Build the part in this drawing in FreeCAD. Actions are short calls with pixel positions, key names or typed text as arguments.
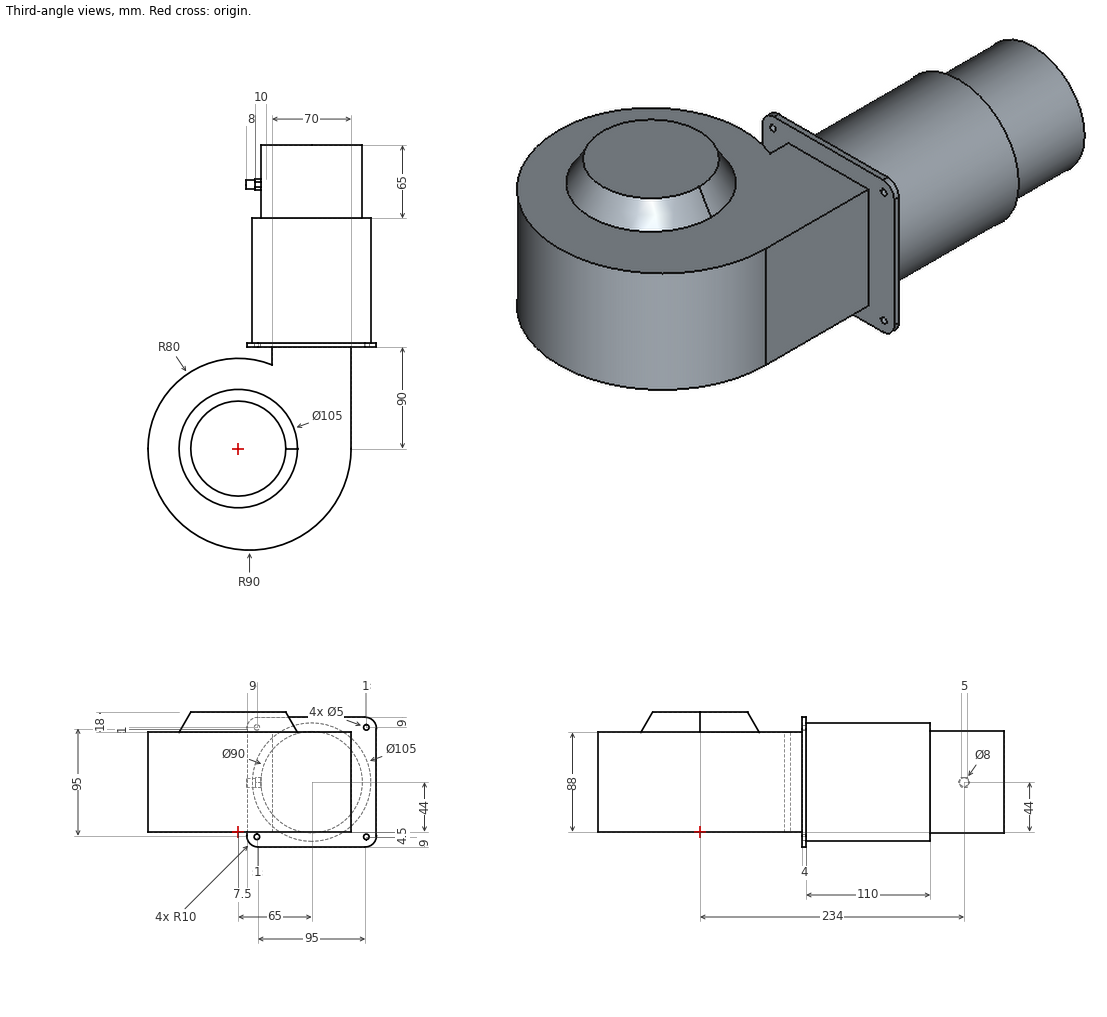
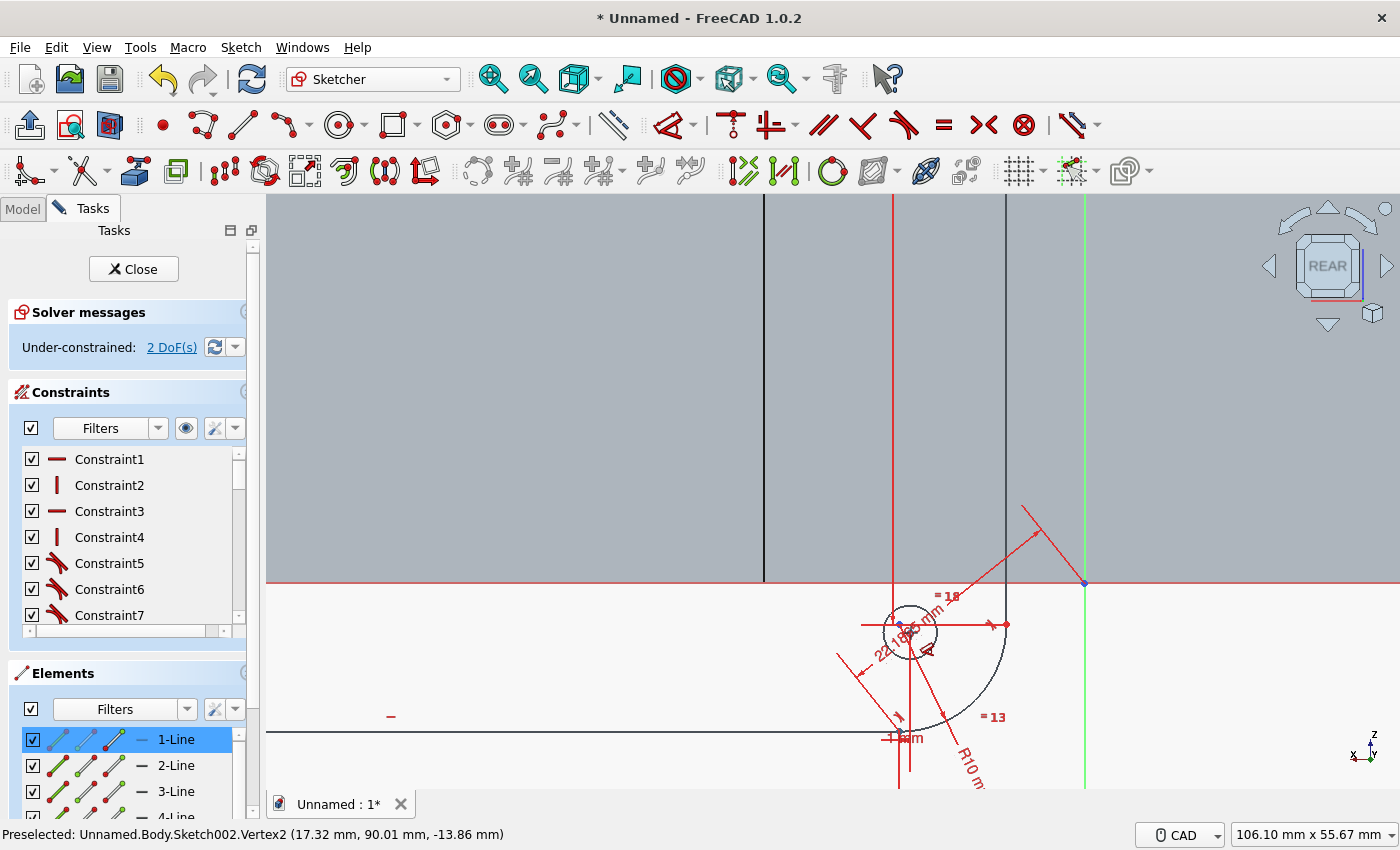
click(910, 632)
click(944, 682)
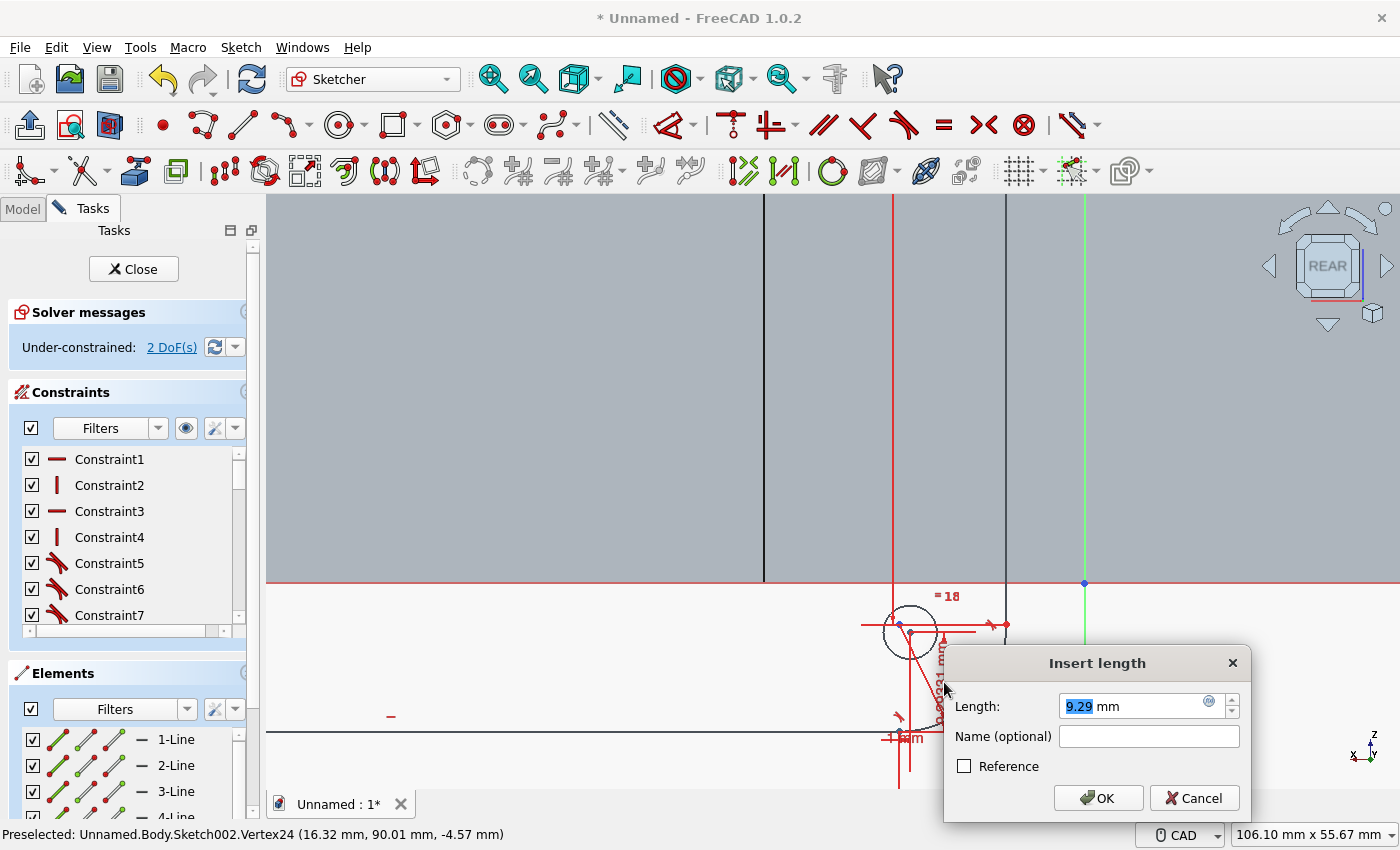
text(9)
key(Return)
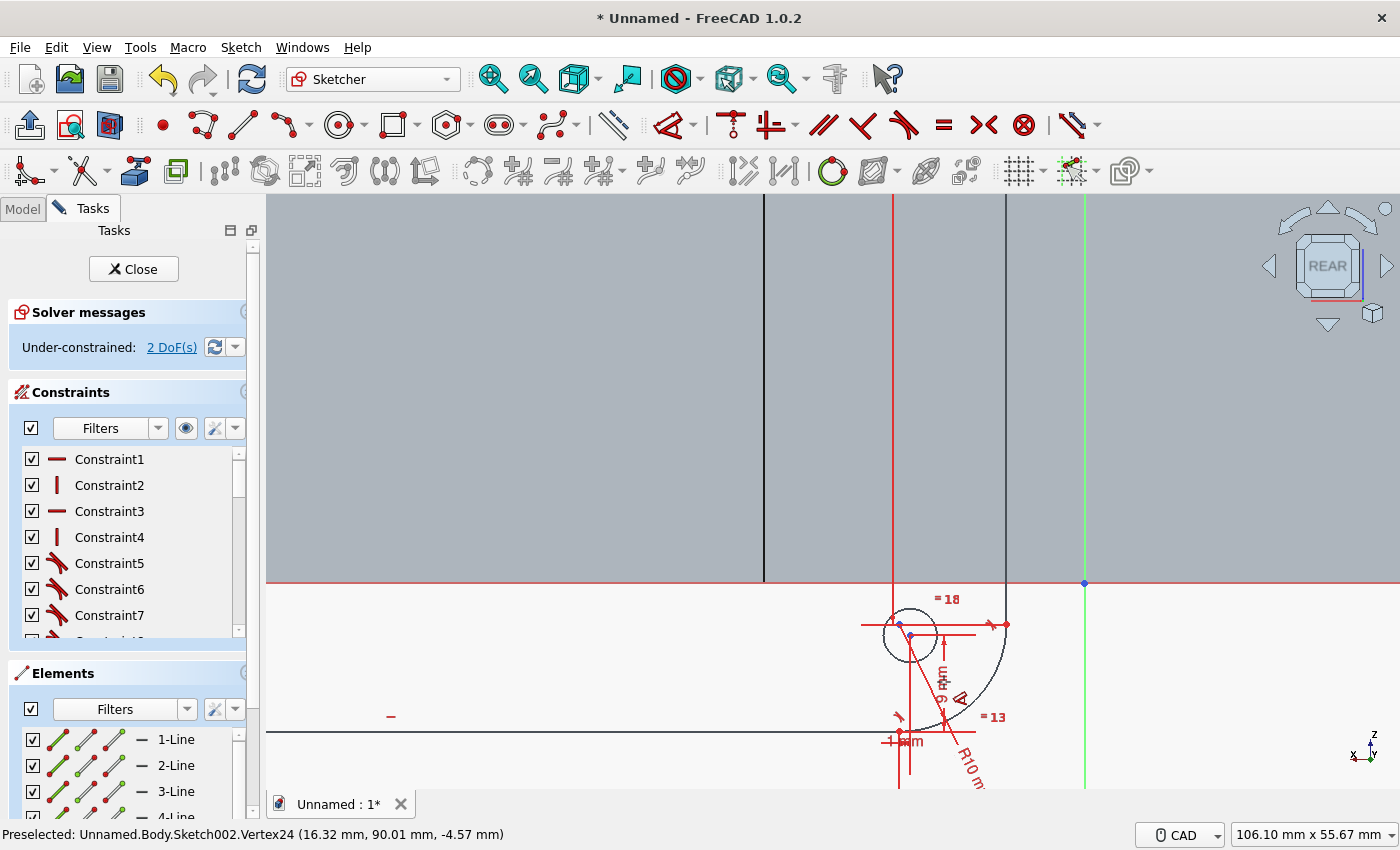
scroll(909, 655, down, 6)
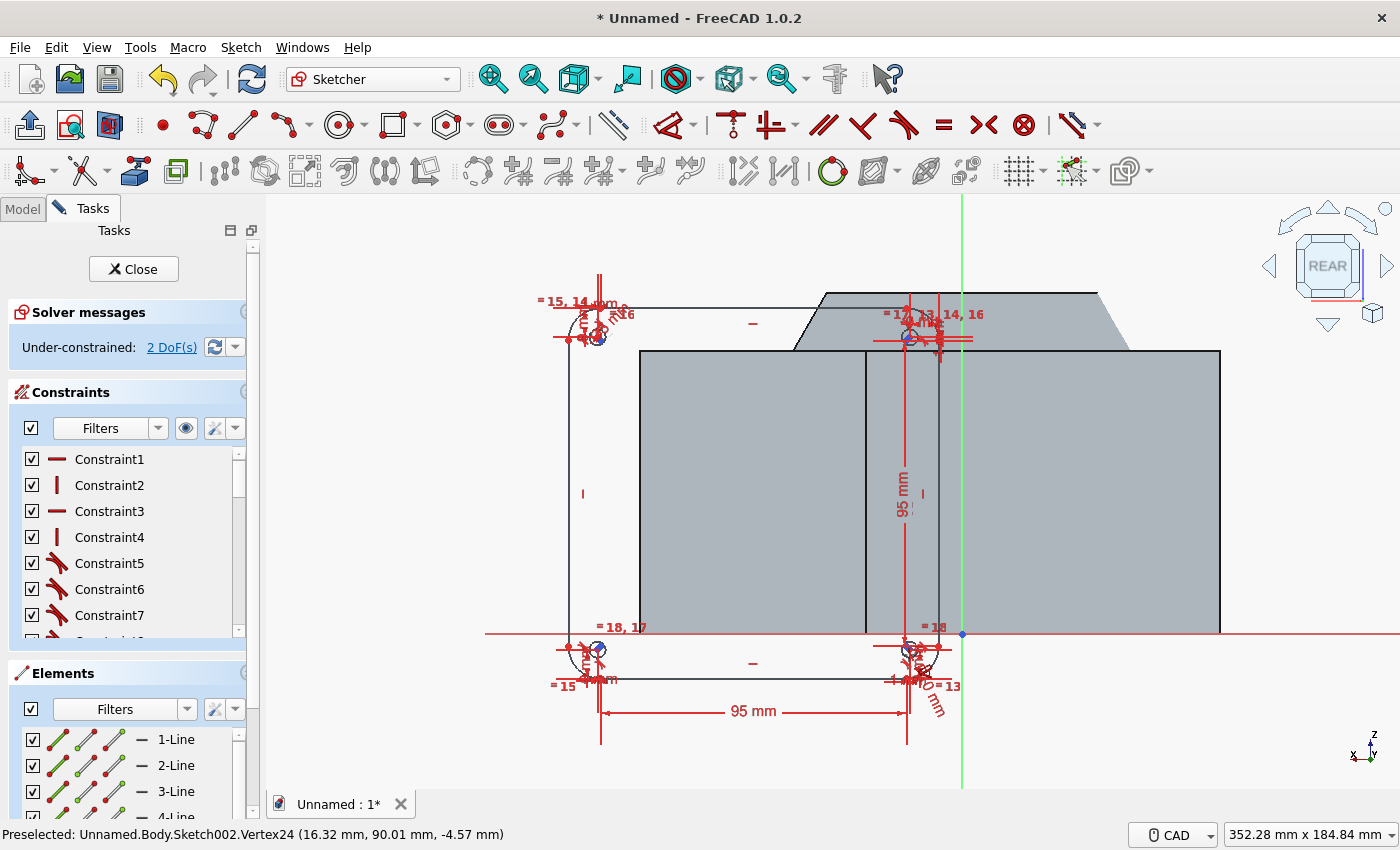
scroll(598, 650, up, 6)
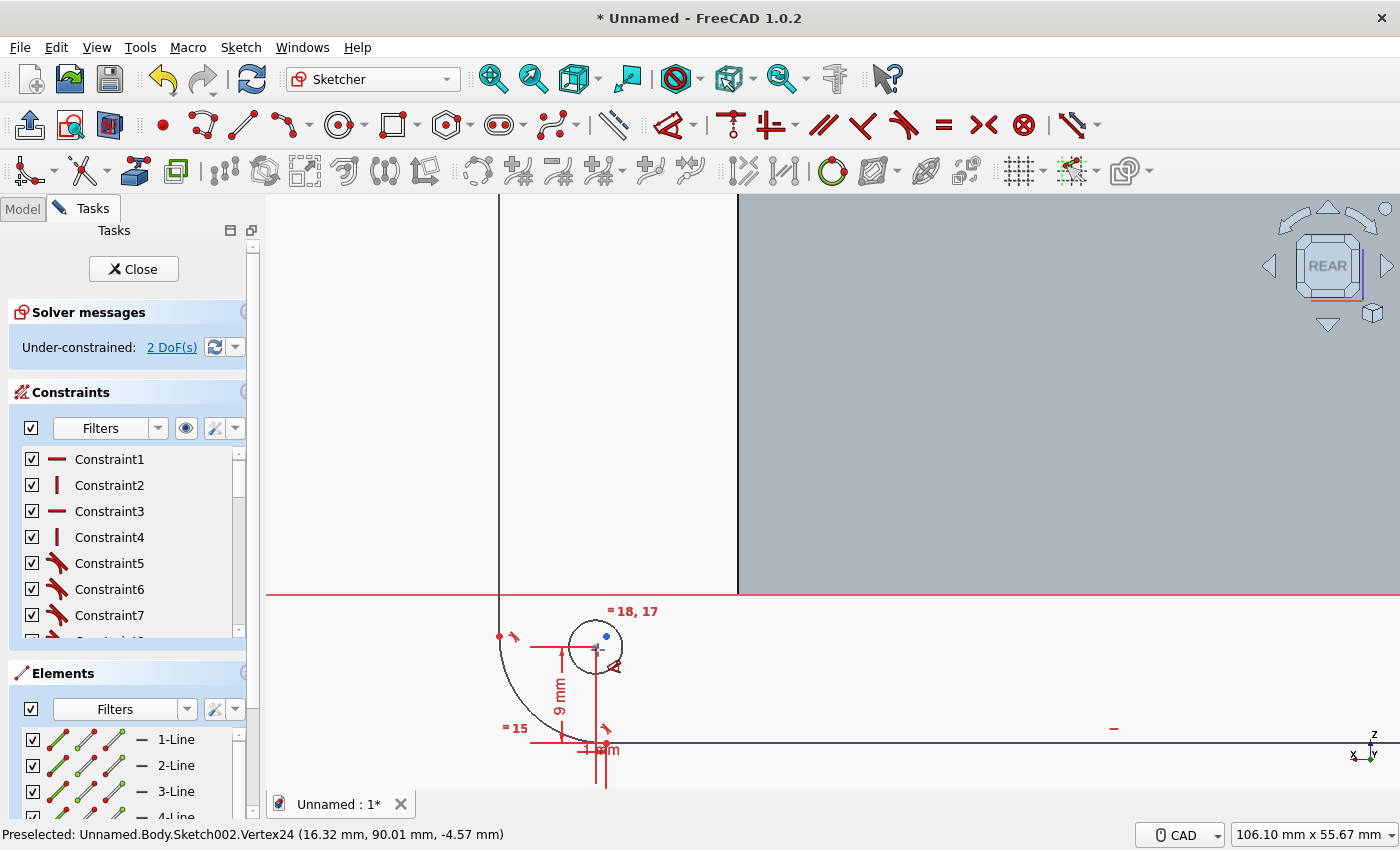
click(596, 647)
click(562, 621)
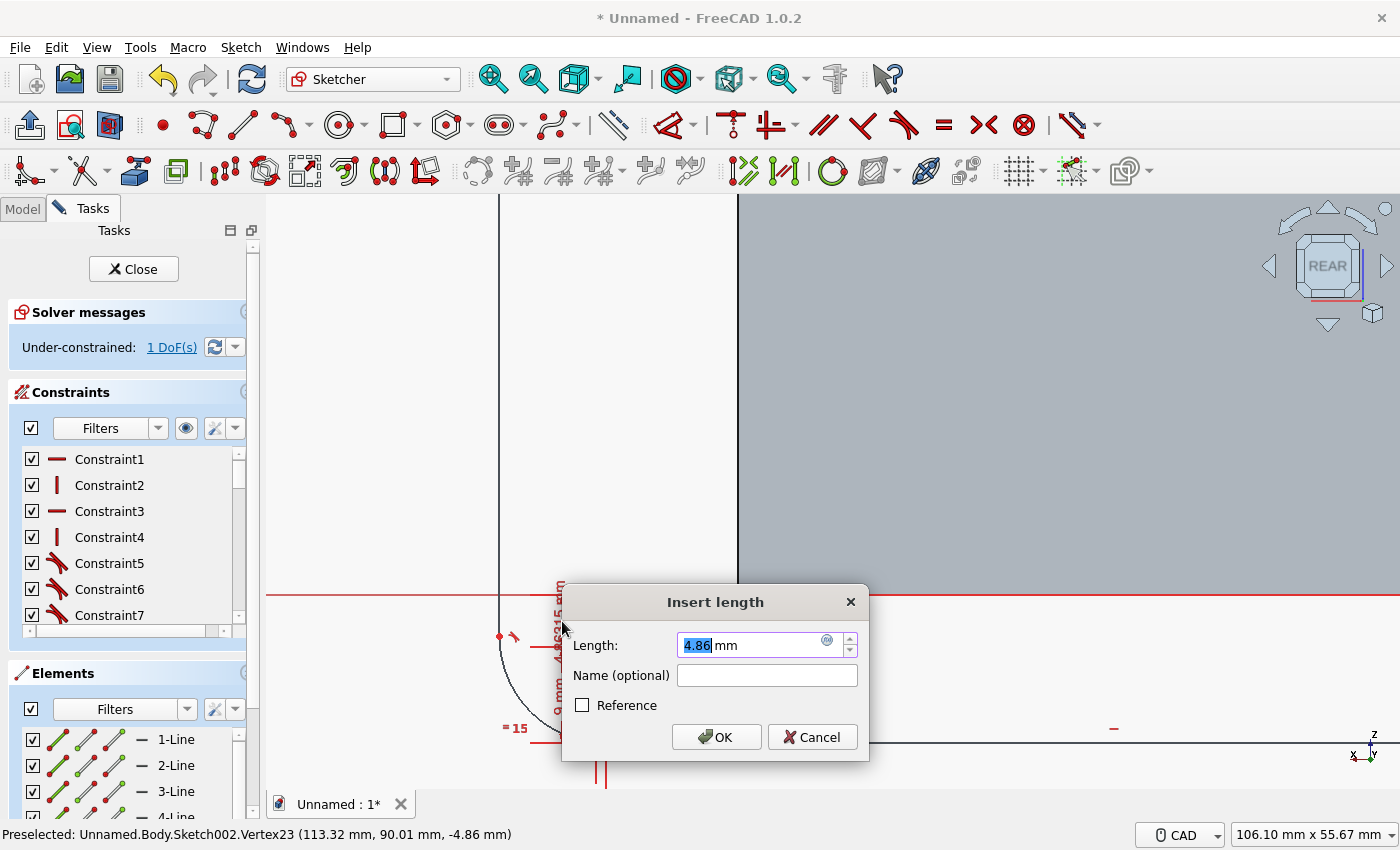
text(4.5)
key(Return)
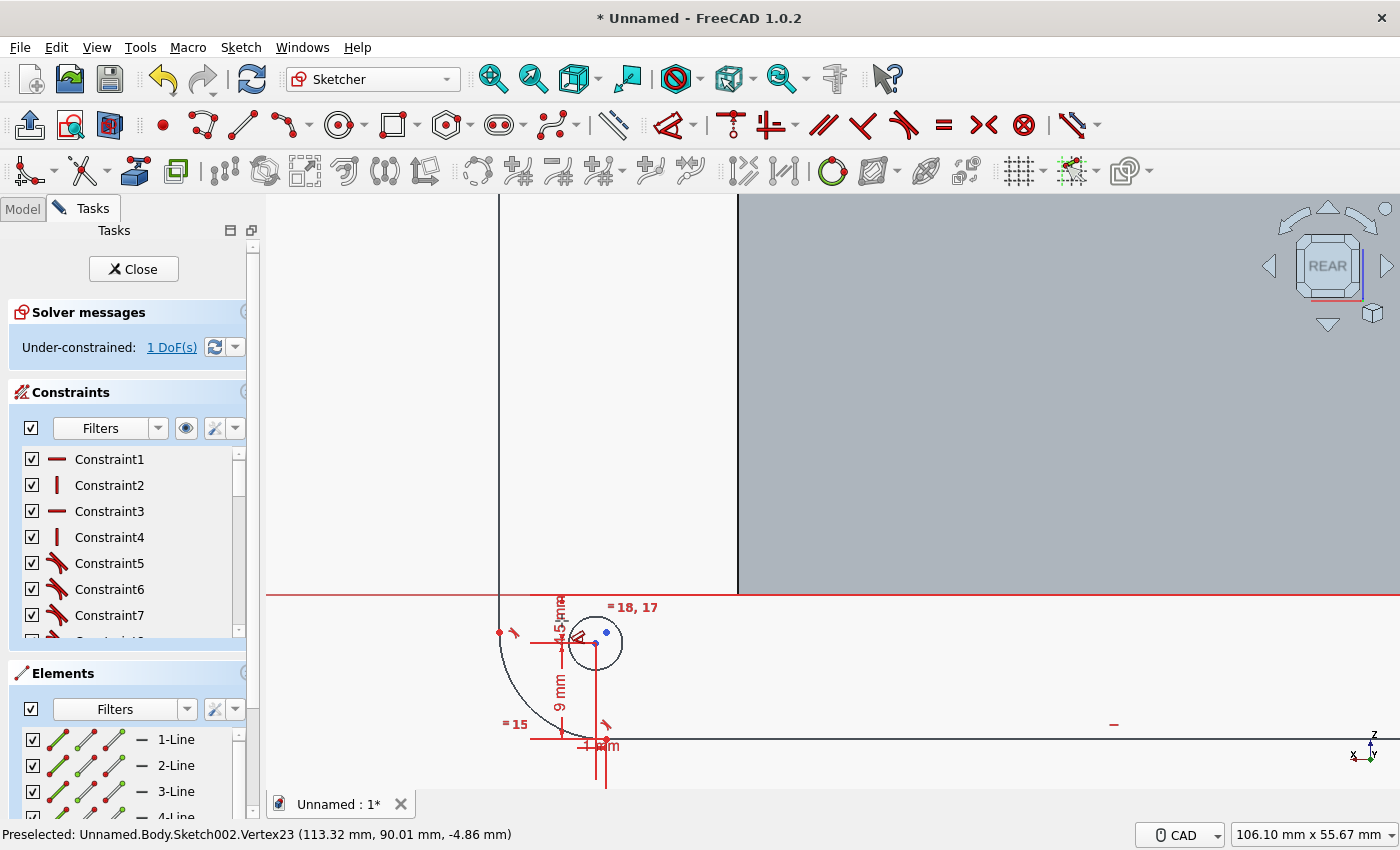
scroll(597, 650, down, 6)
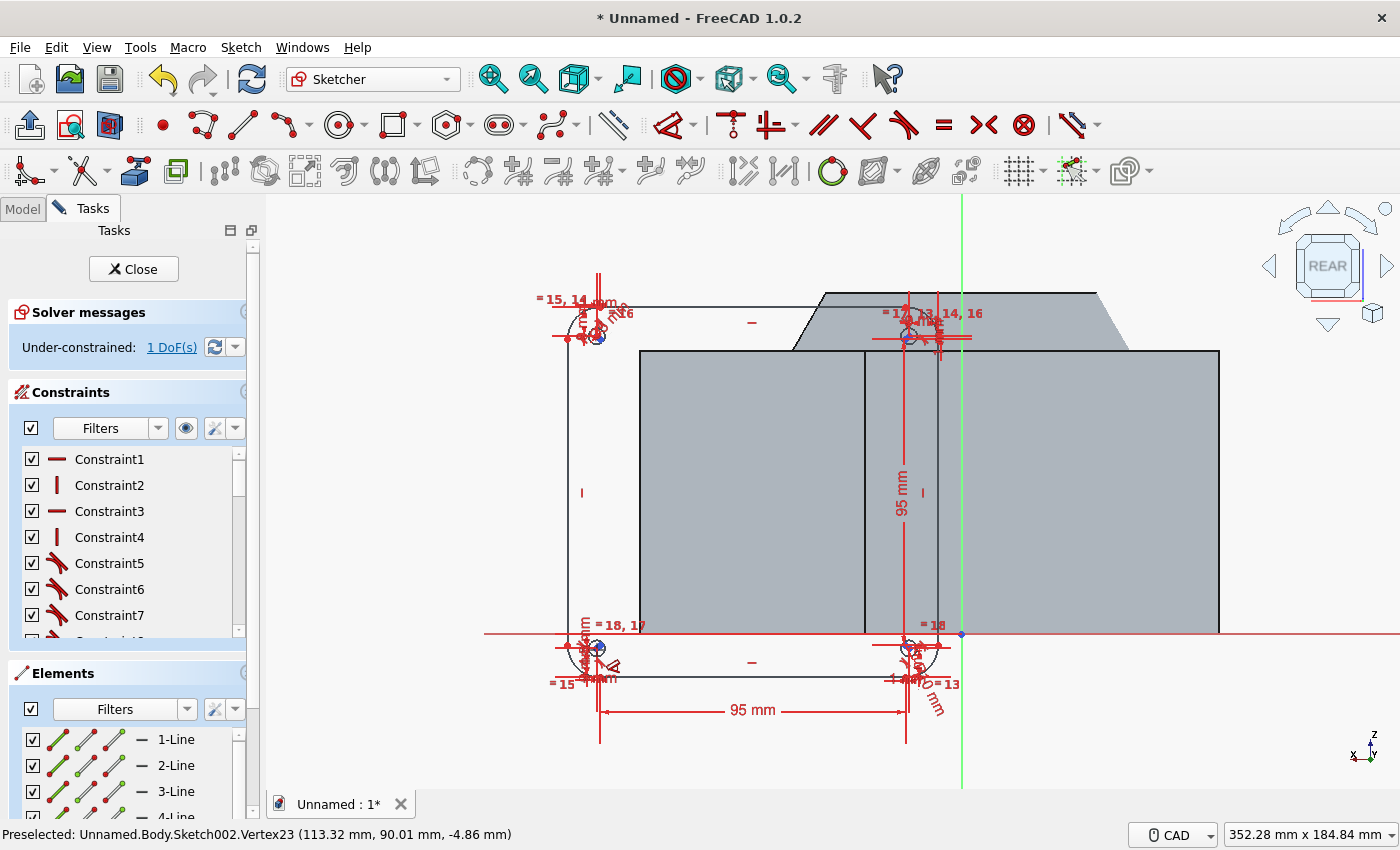
scroll(938, 645, up, 3)